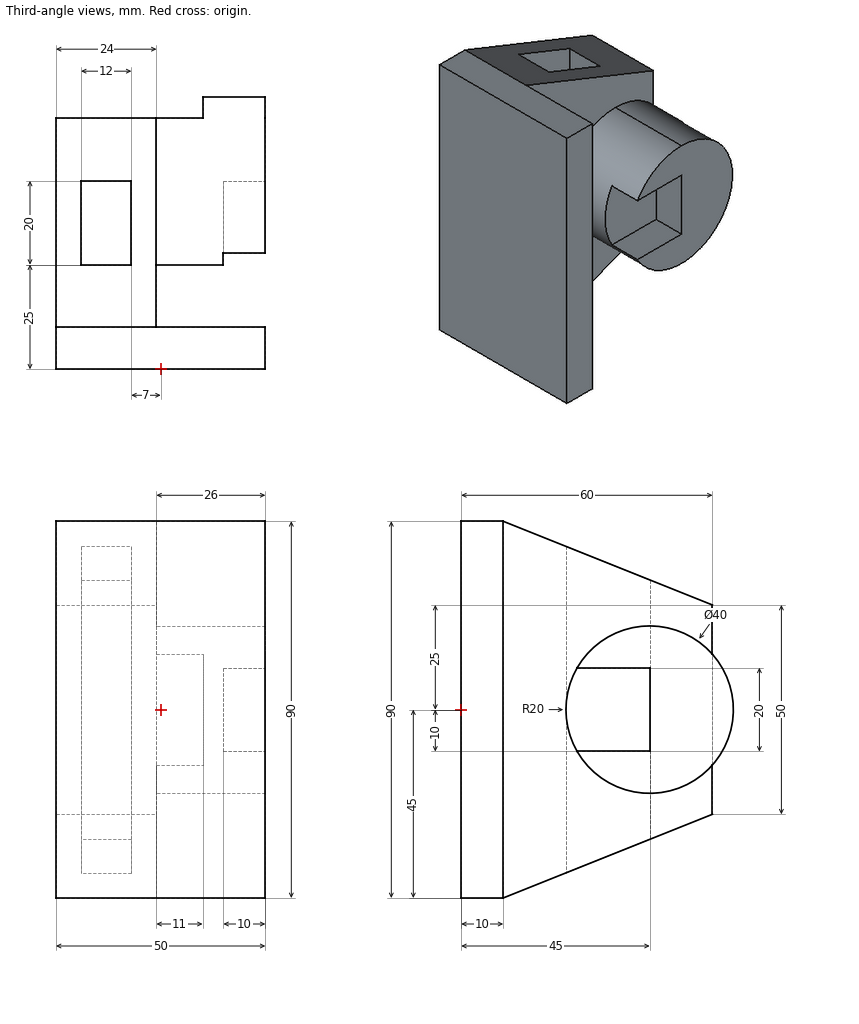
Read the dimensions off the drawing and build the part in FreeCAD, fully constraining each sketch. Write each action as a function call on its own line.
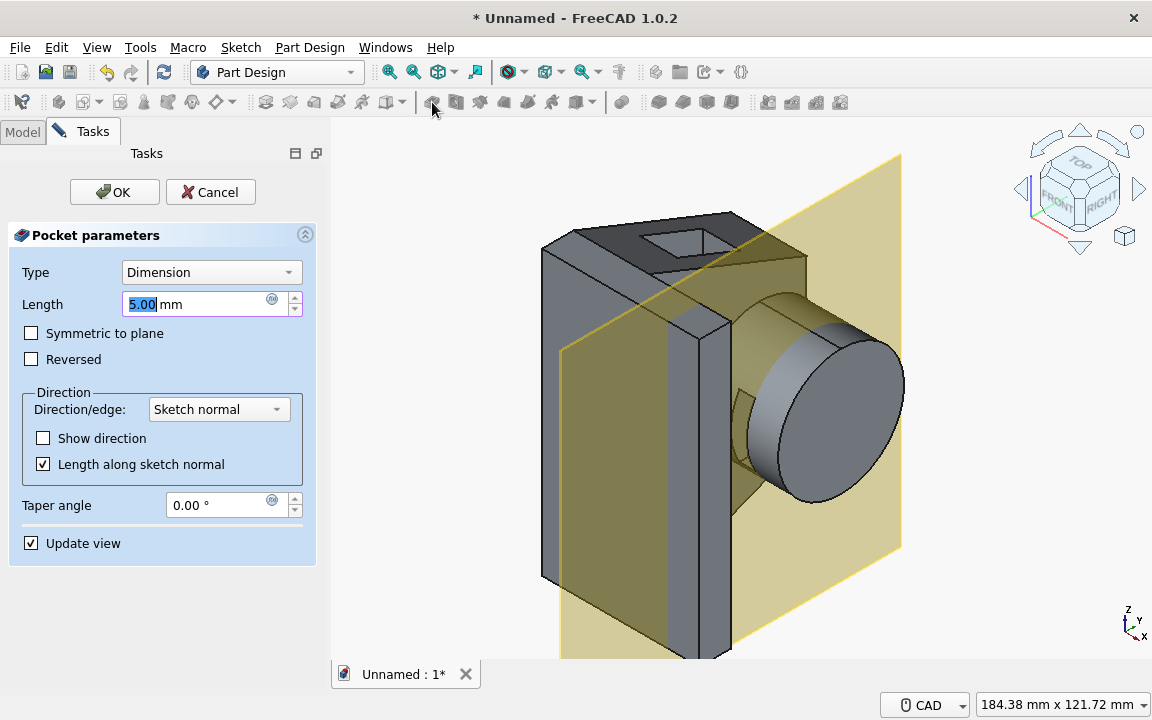
text(10)
key(Tab)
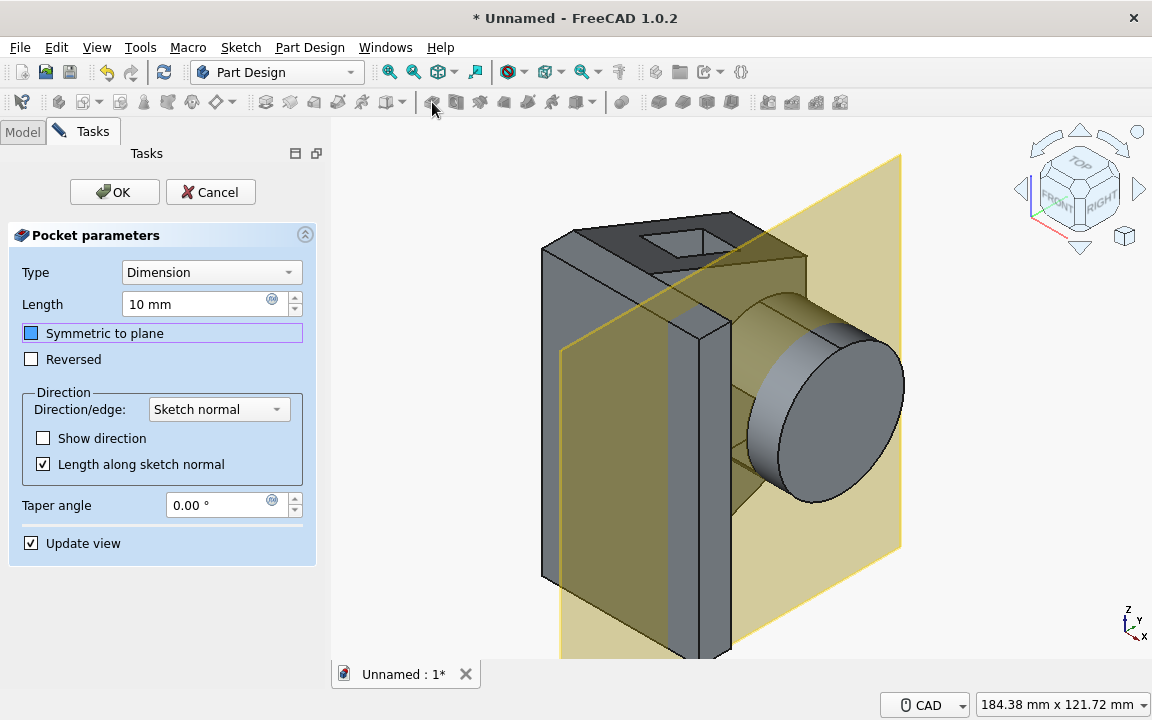
click(30, 359)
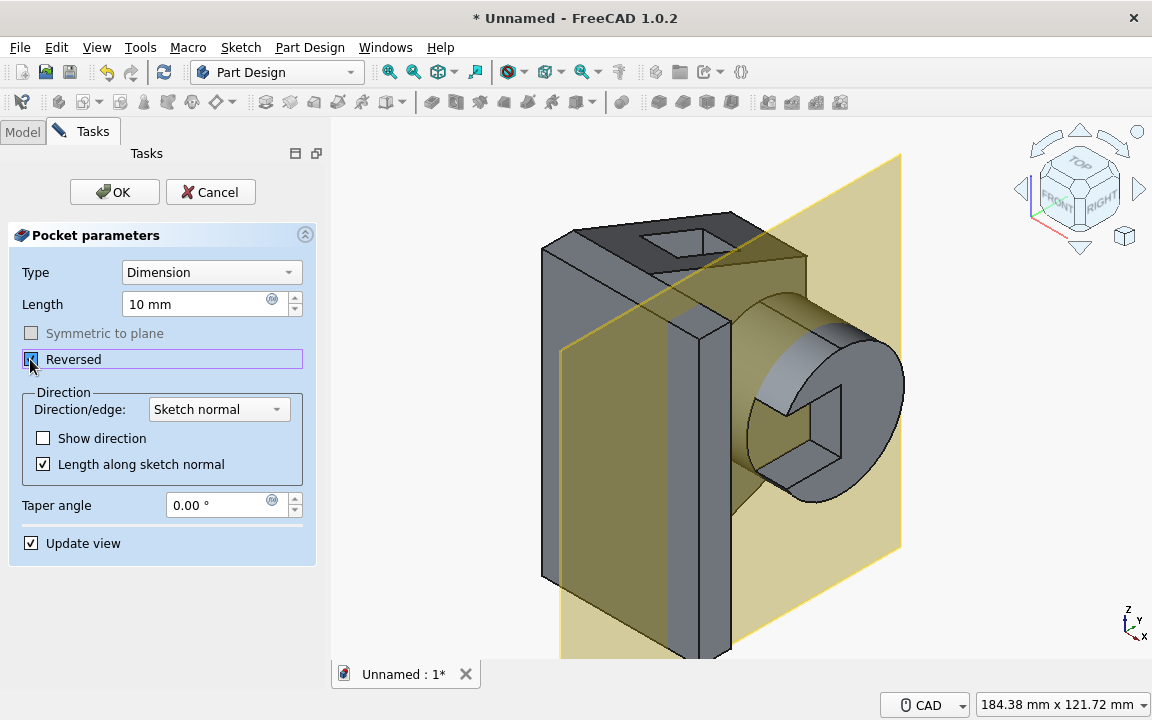
click(115, 192)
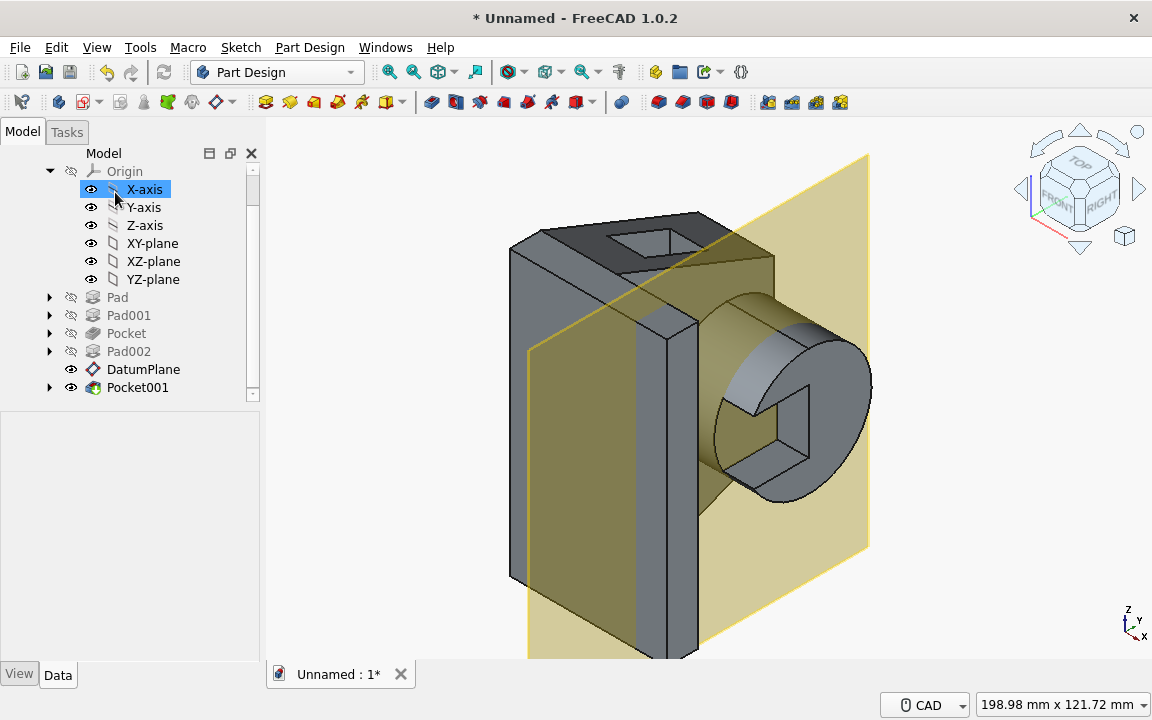
click(116, 369)
key(space)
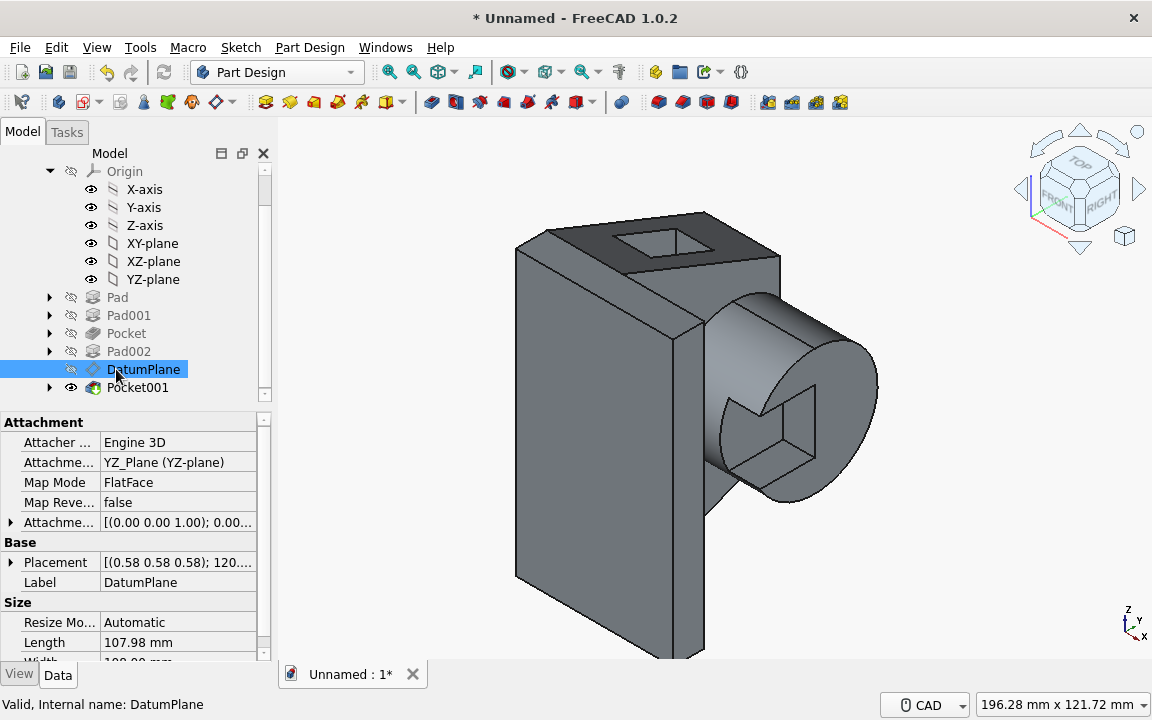
click(390, 72)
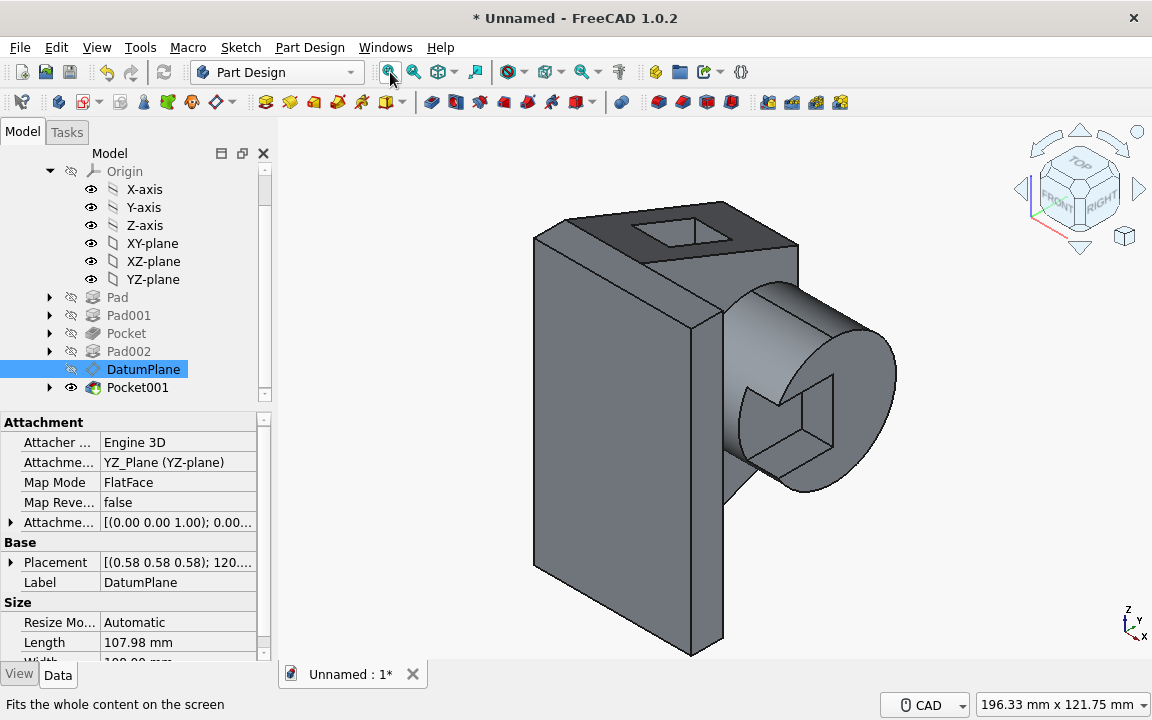
click(720, 287)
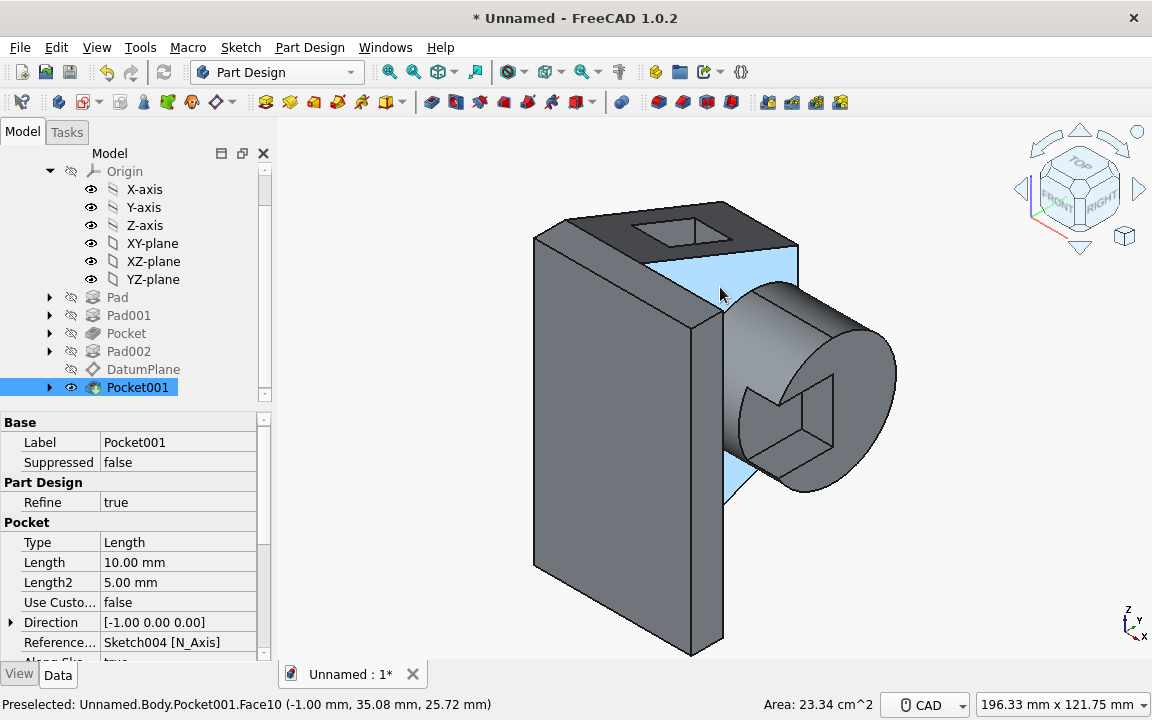
click(84, 102)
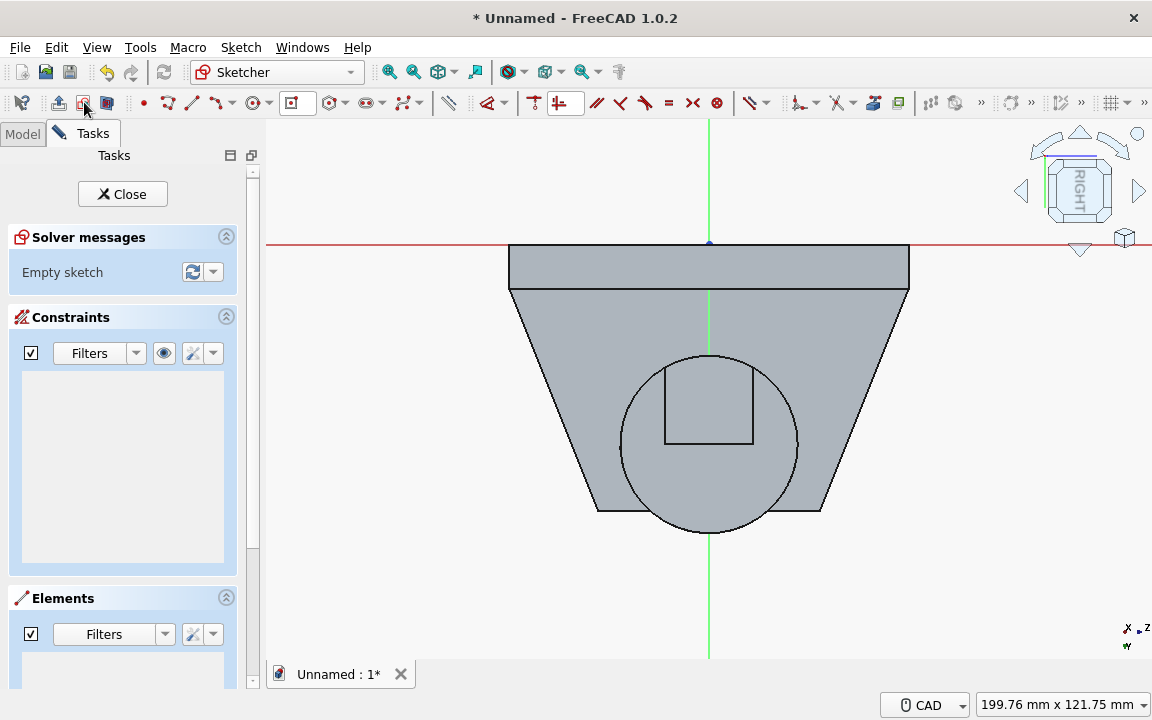
click(192, 104)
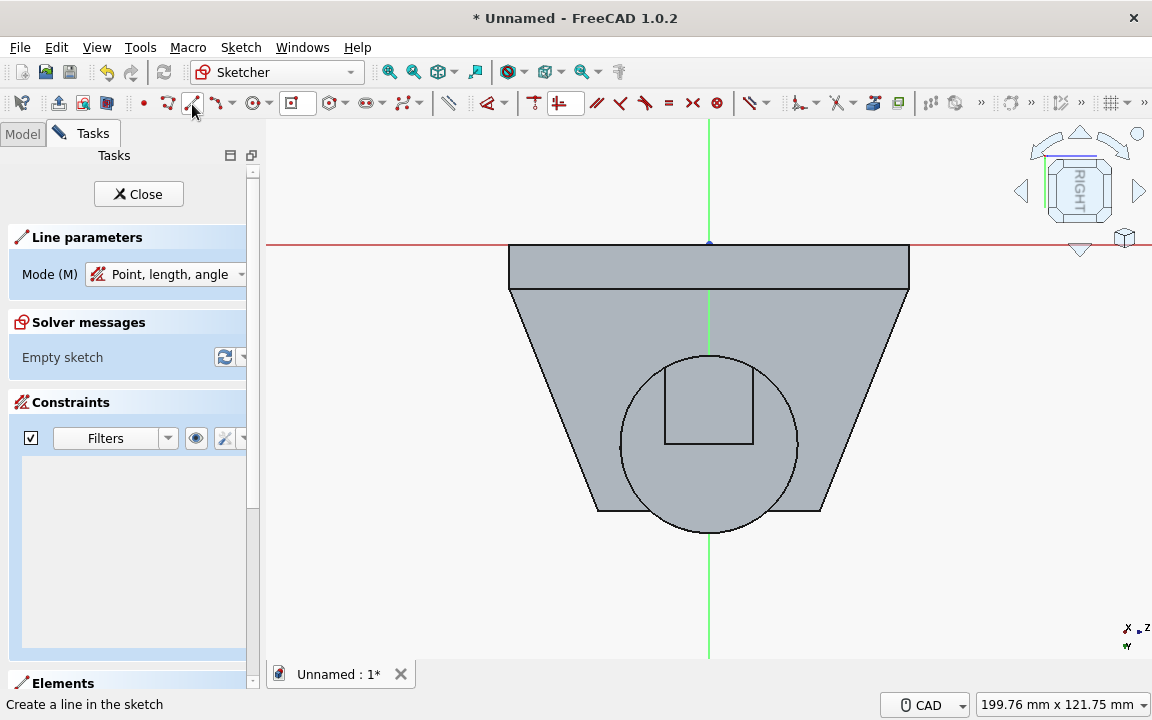
click(650, 511)
click(768, 511)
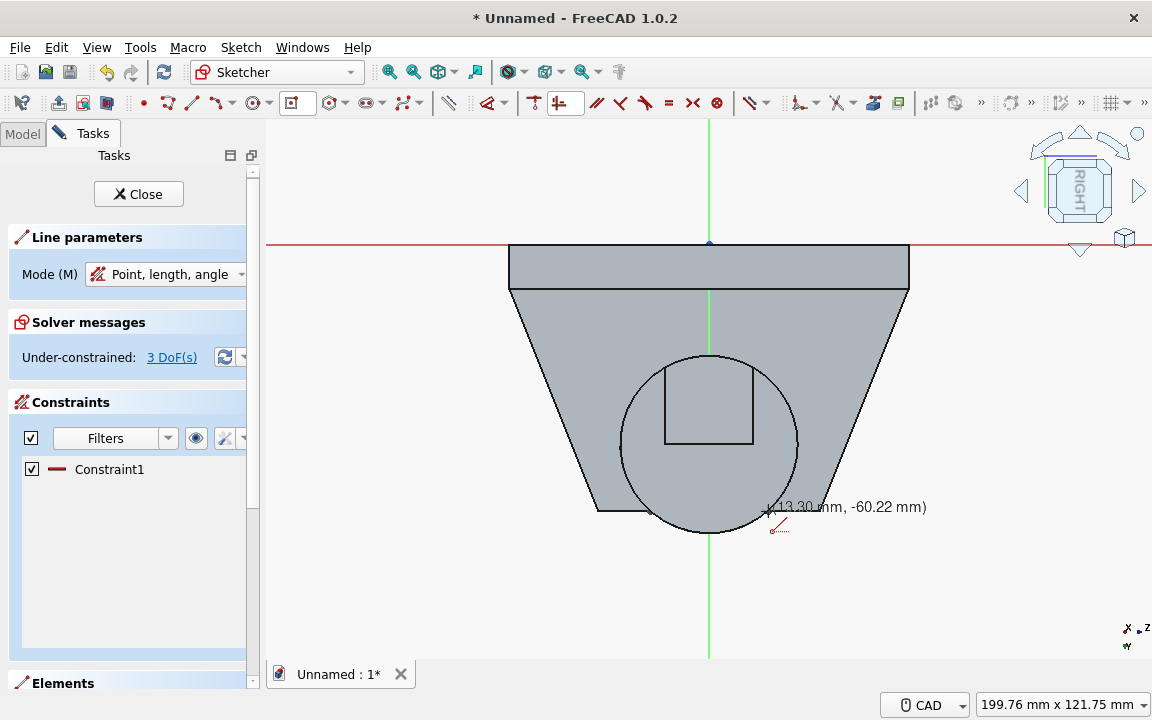
click(216, 104)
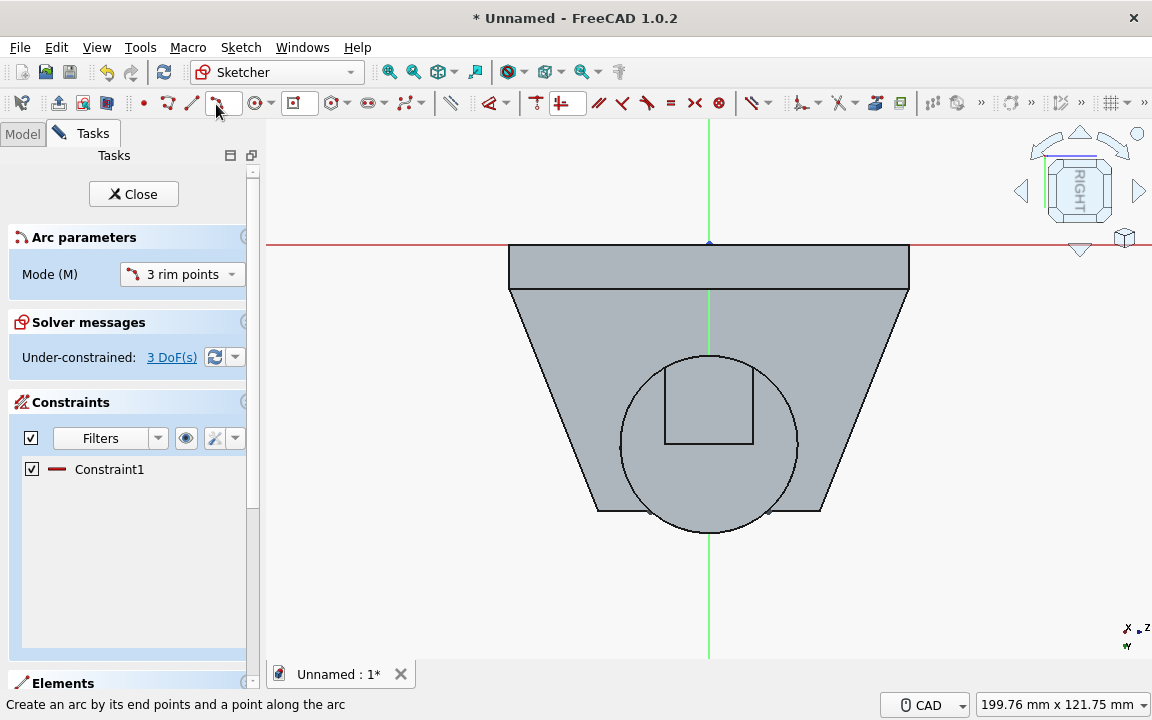
click(768, 512)
click(650, 512)
click(684, 530)
key(Escape)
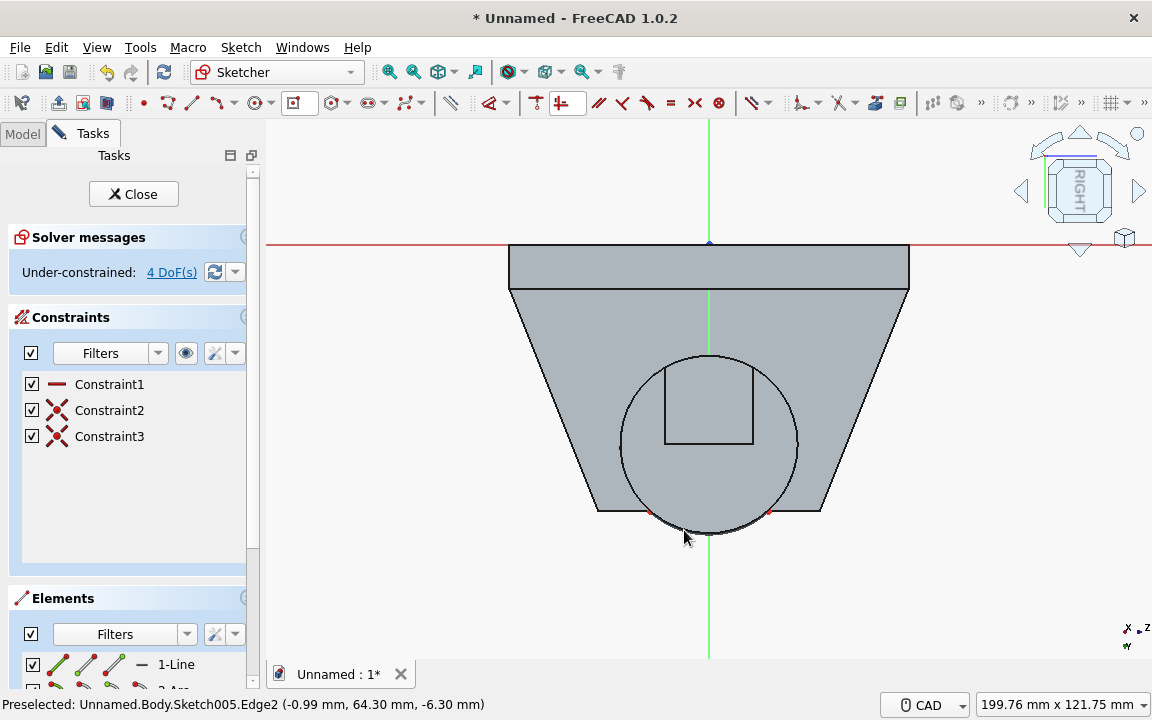
click(709, 446)